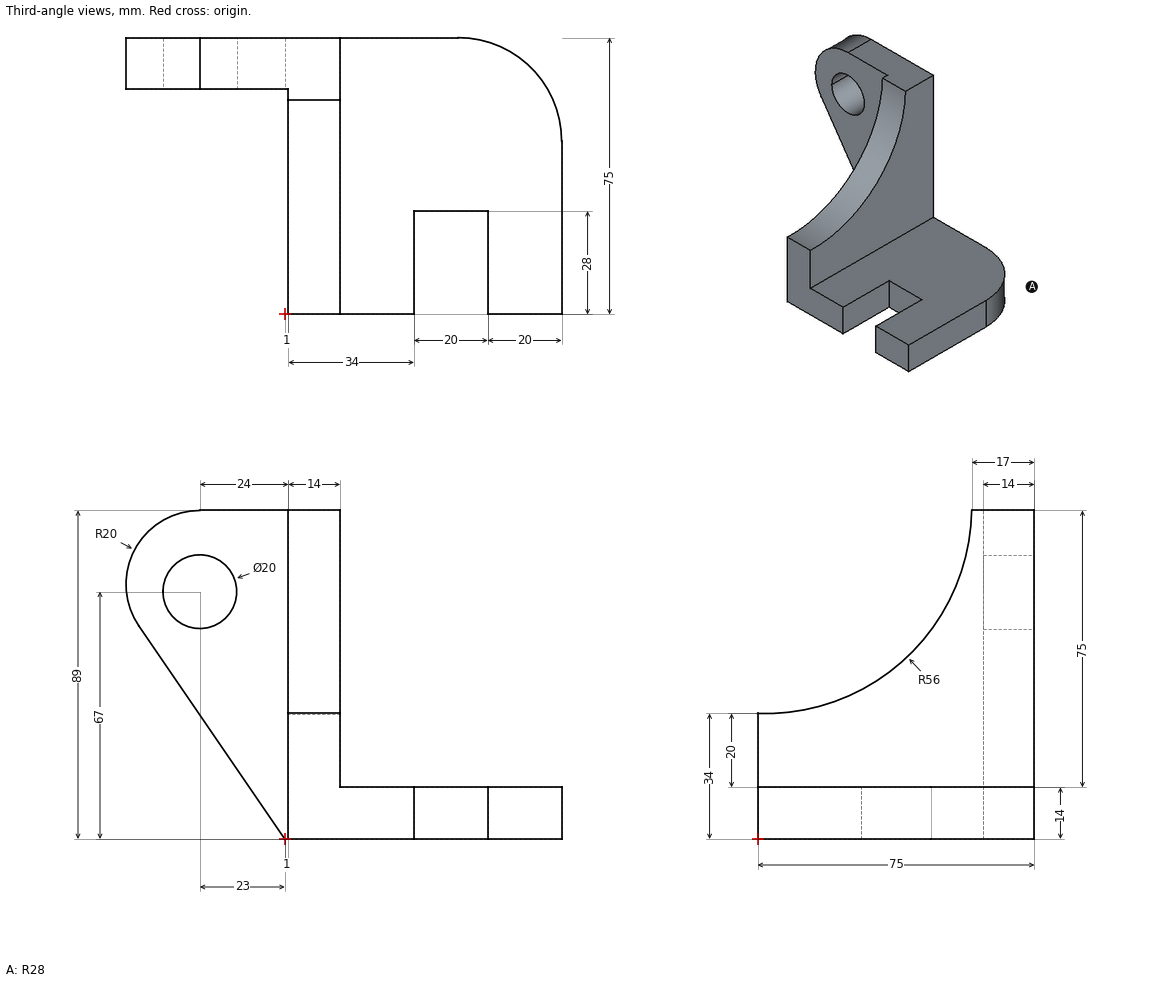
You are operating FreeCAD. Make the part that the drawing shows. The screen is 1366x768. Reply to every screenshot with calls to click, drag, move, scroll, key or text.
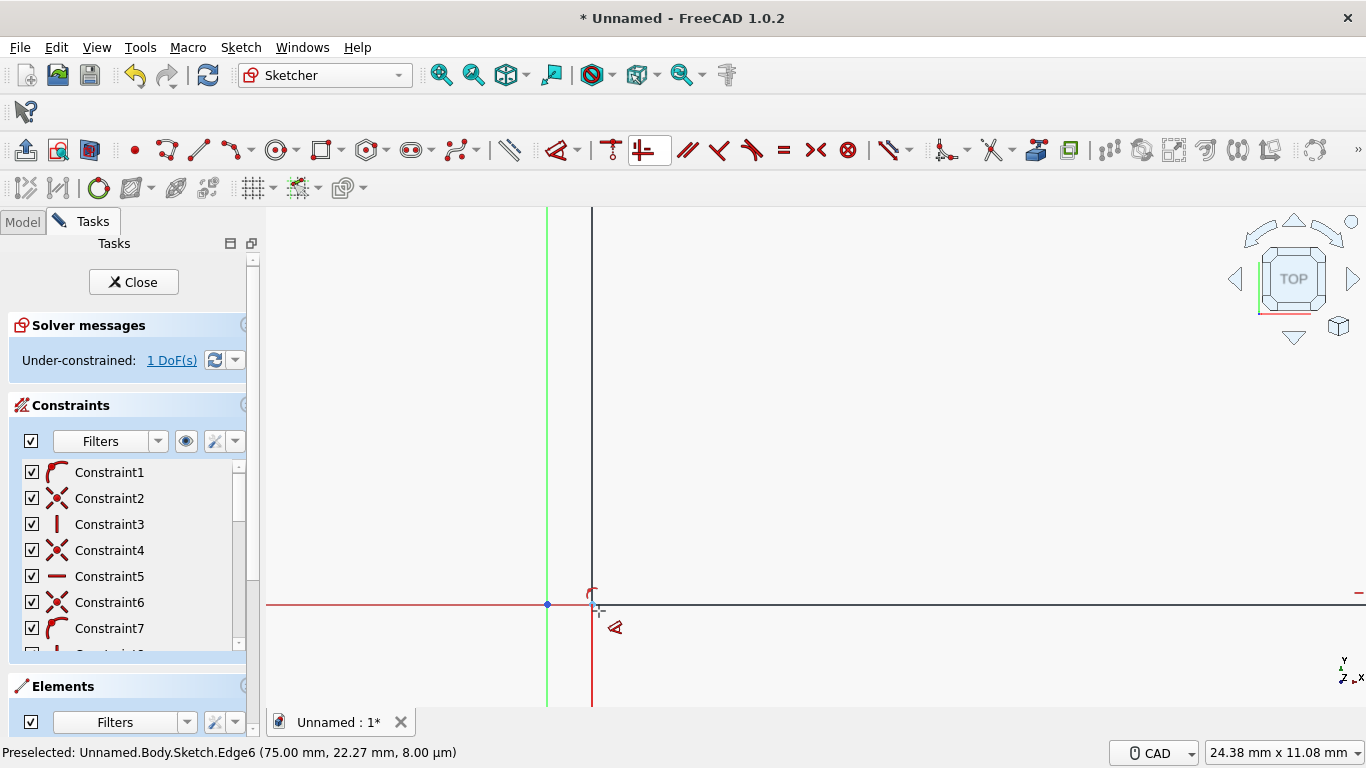
click(592, 605)
click(570, 639)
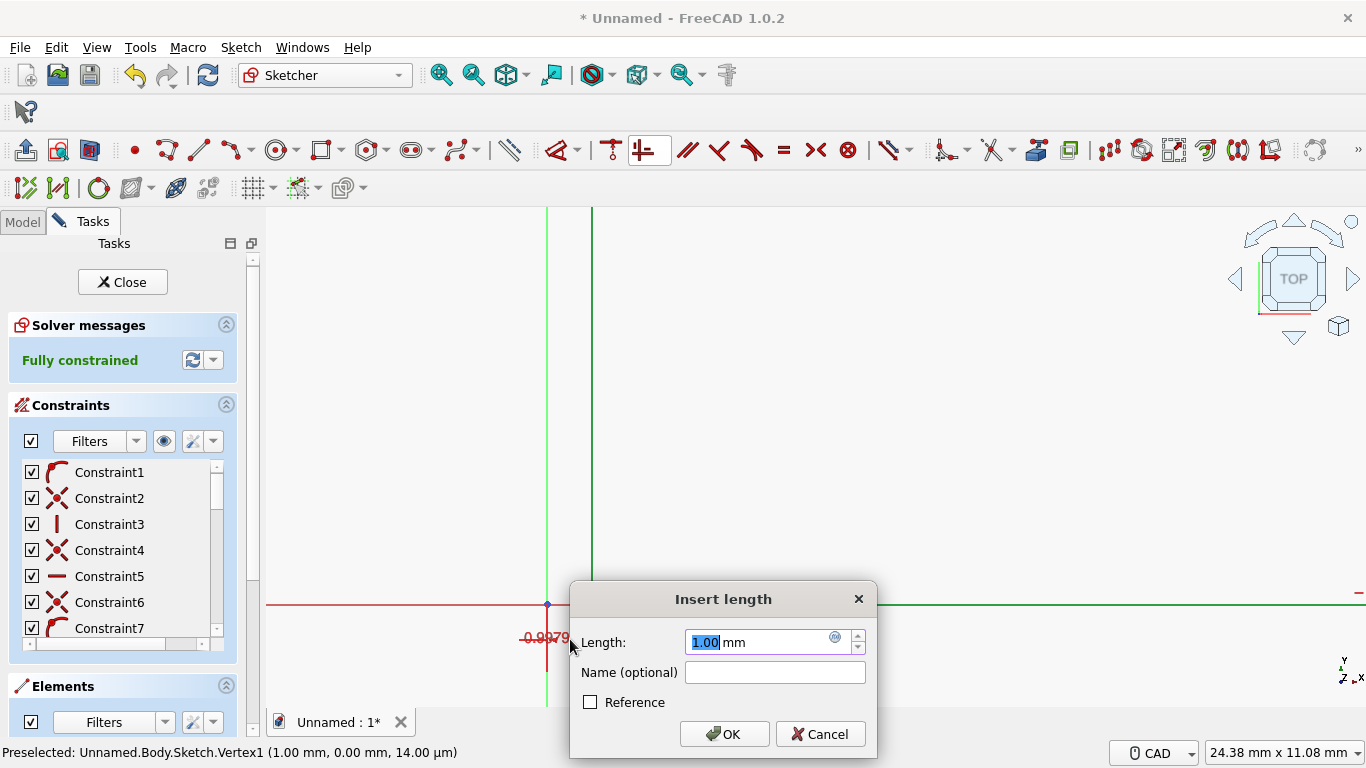
text(1)
key(Return)
key(Escape)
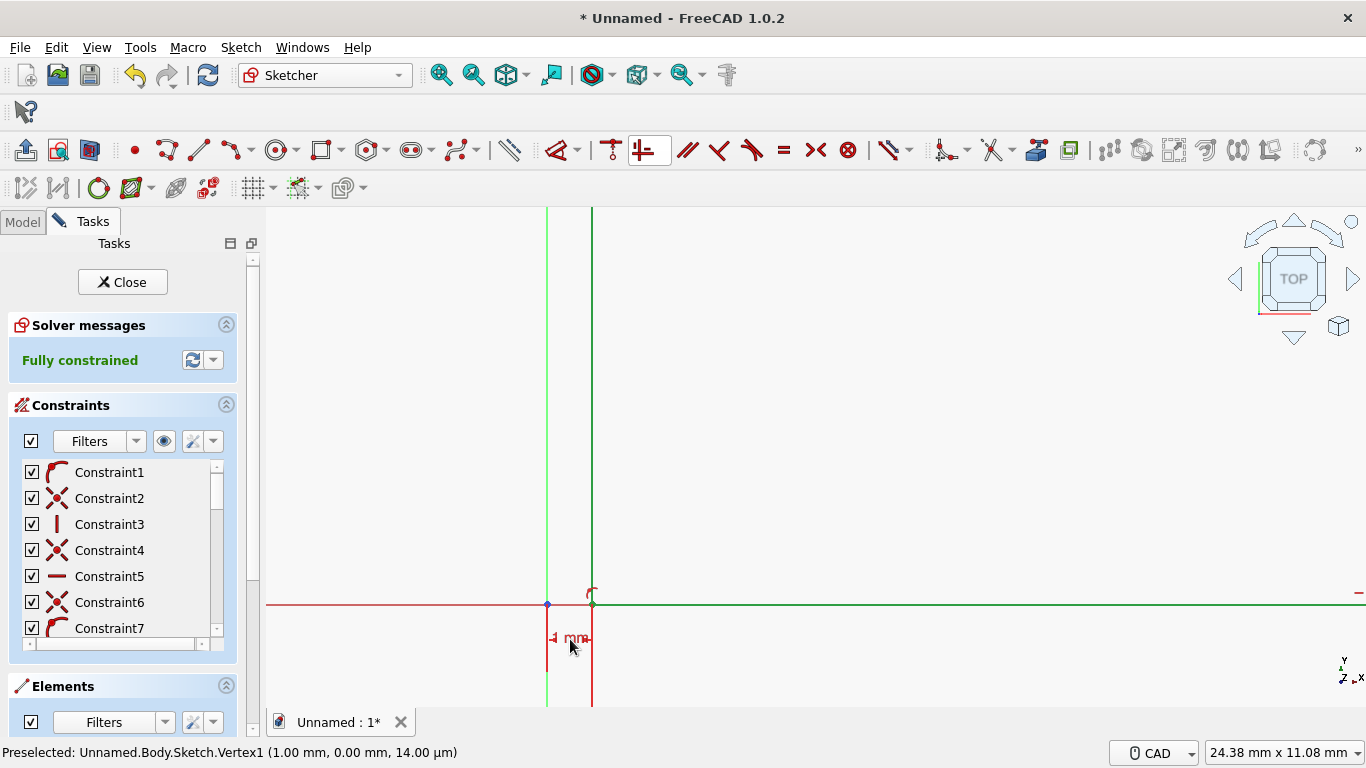
click(123, 282)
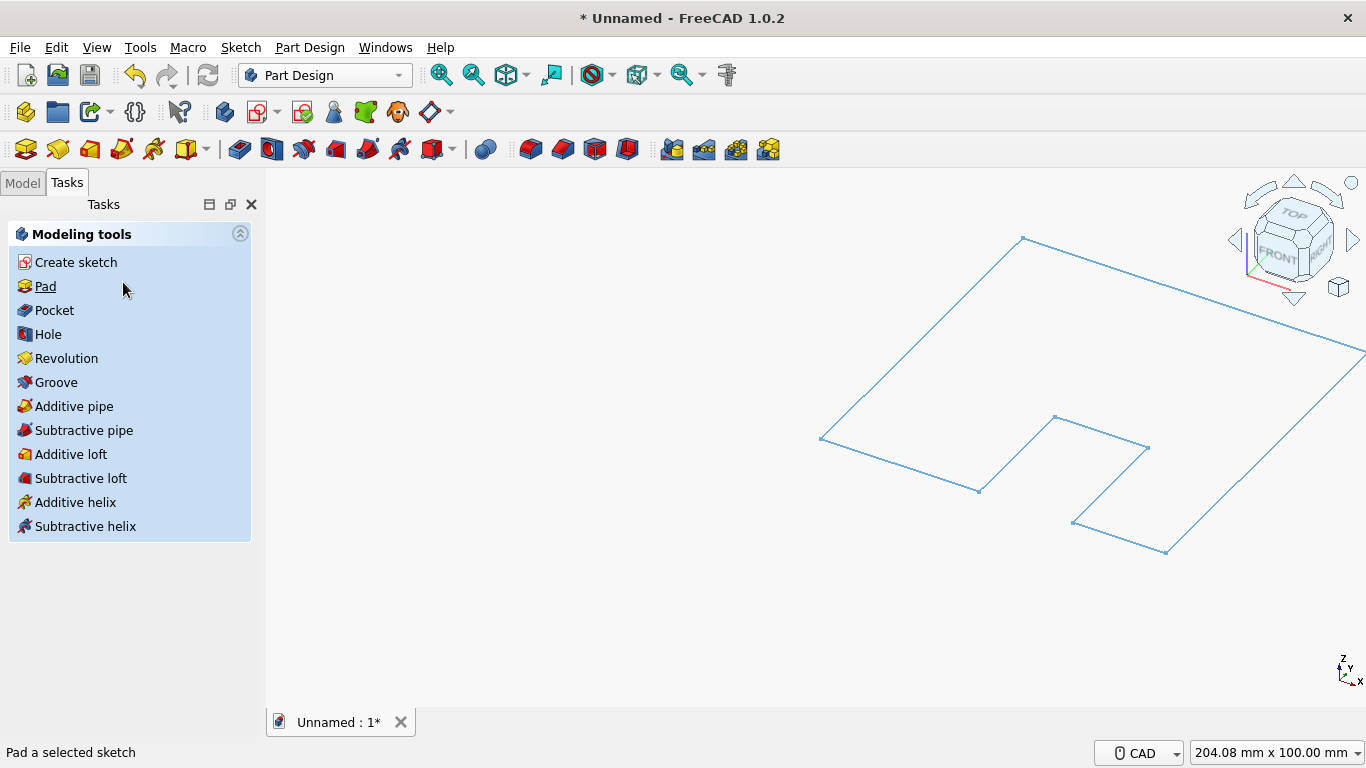
click(26, 150)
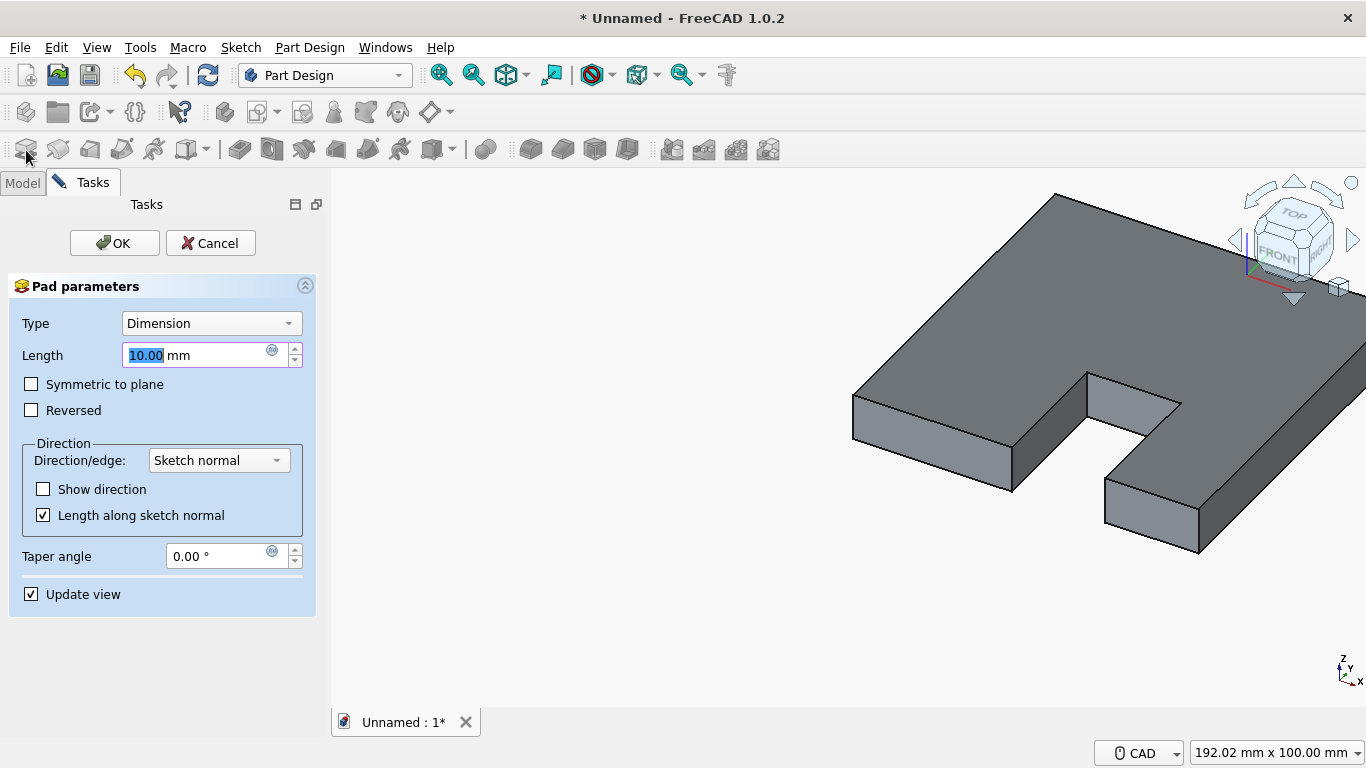
text(14)
key(Tab)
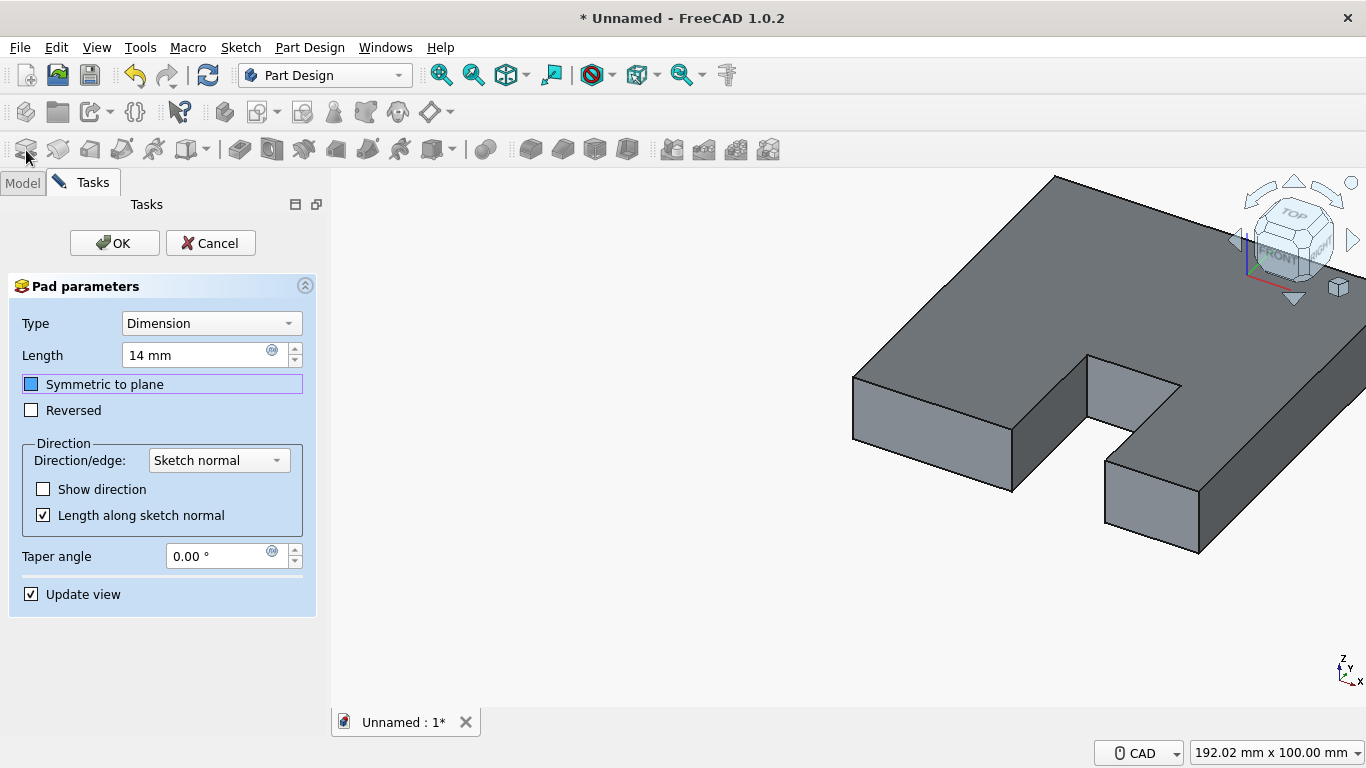
click(115, 243)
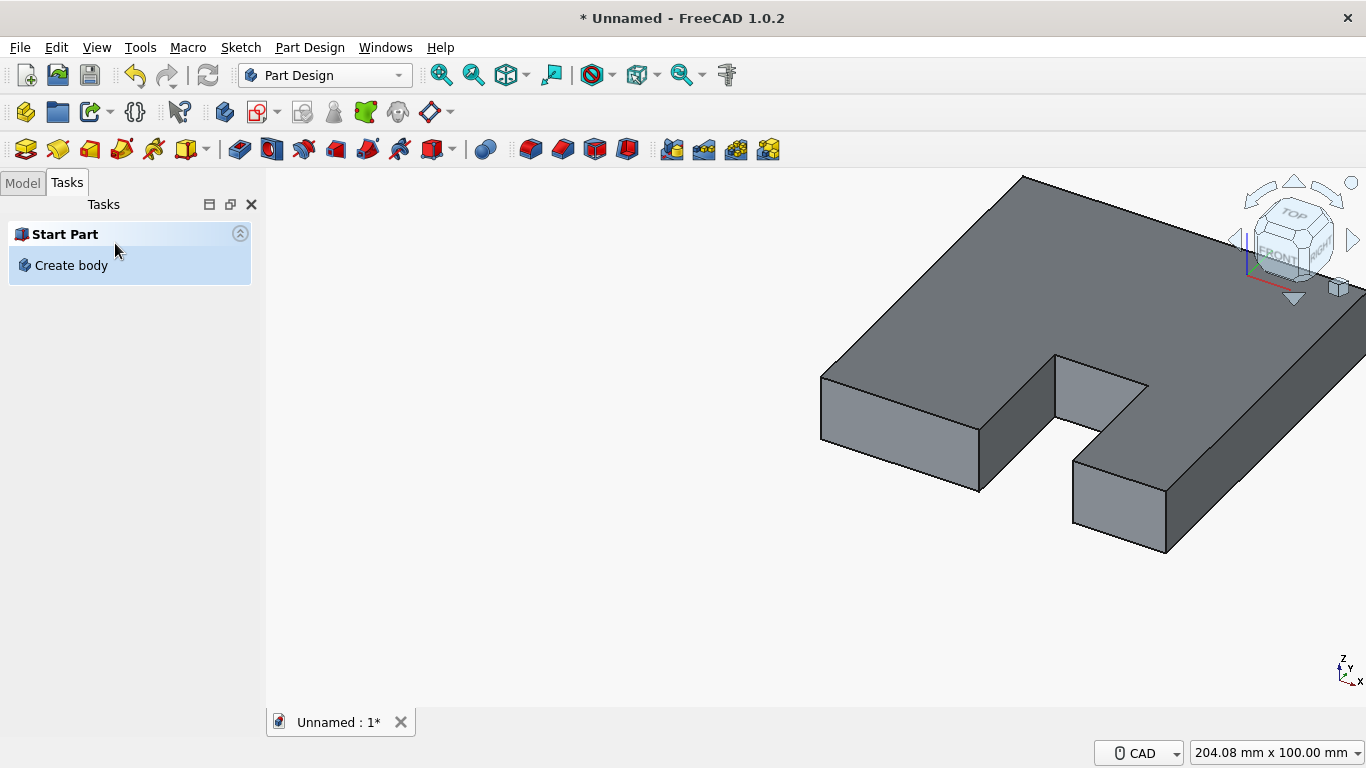
click(442, 76)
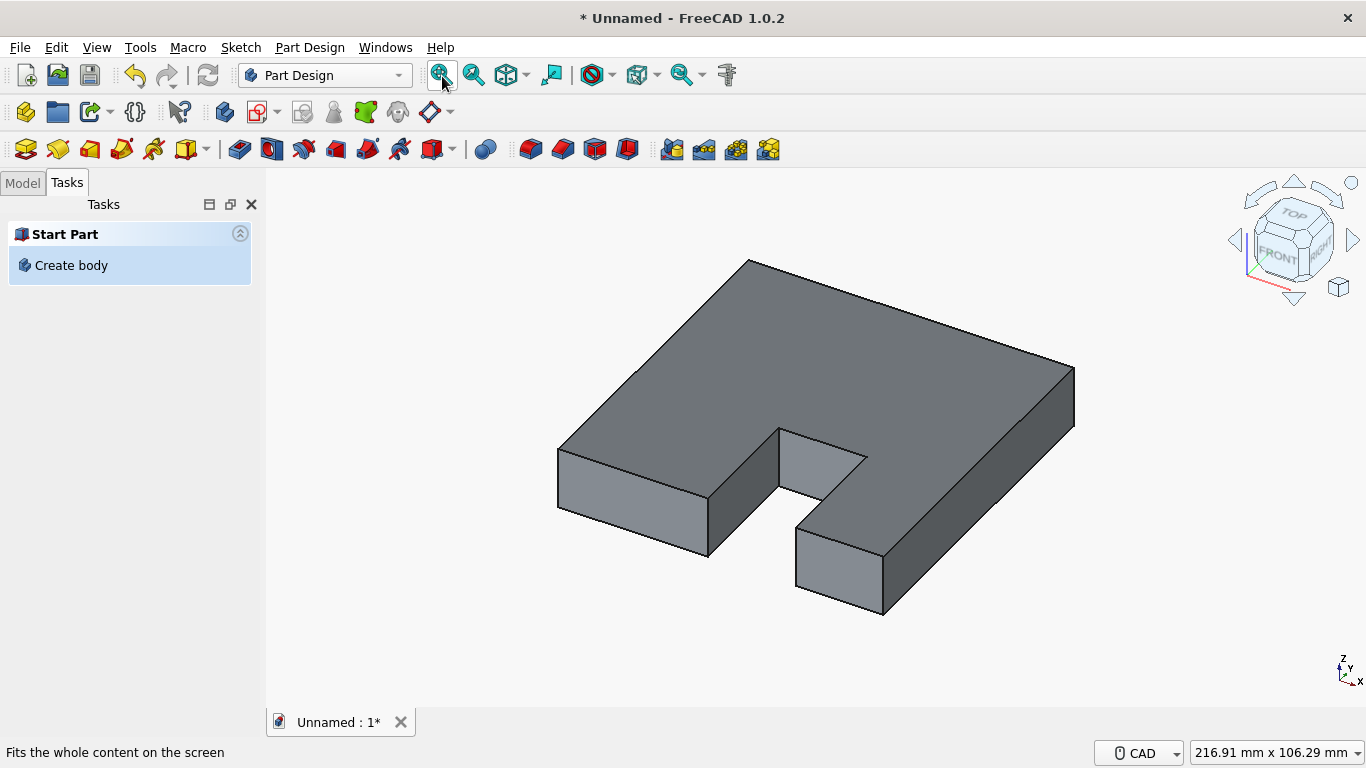
key(6)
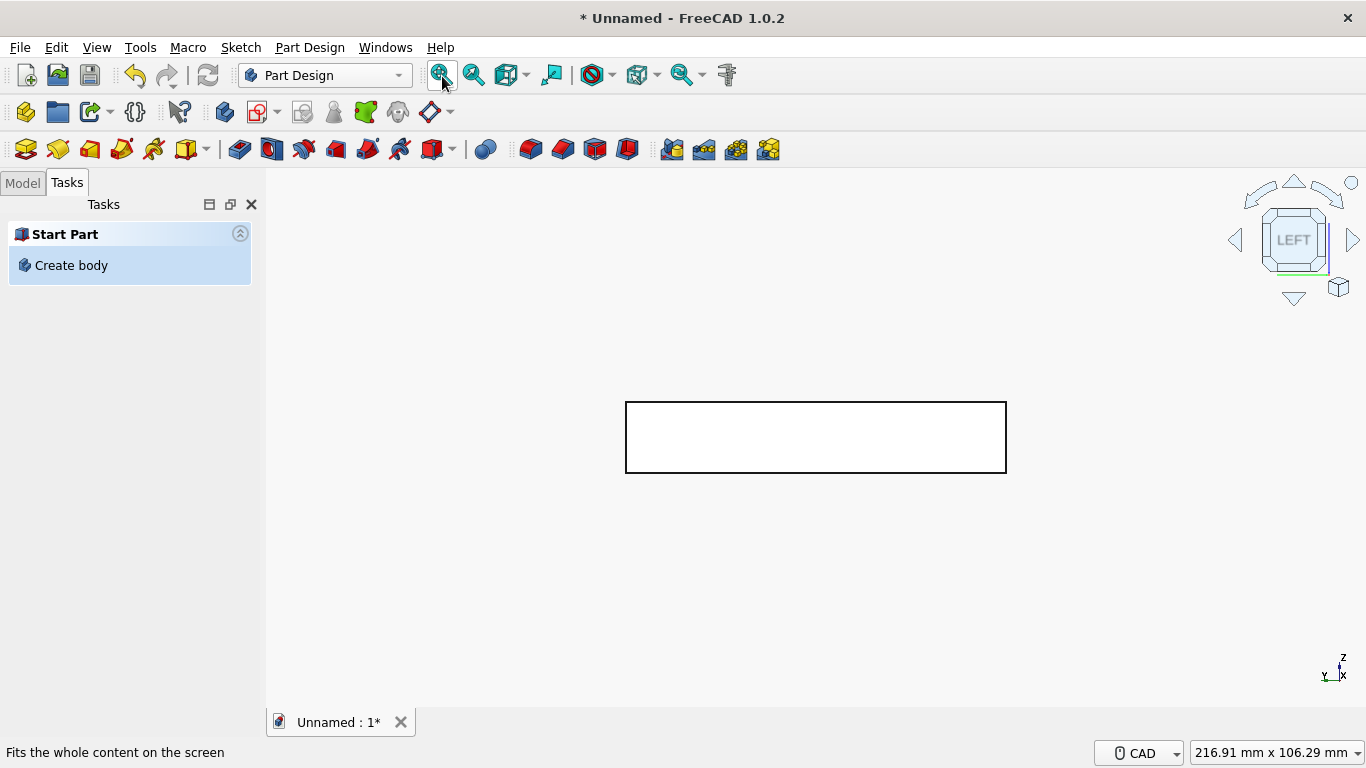
click(442, 76)